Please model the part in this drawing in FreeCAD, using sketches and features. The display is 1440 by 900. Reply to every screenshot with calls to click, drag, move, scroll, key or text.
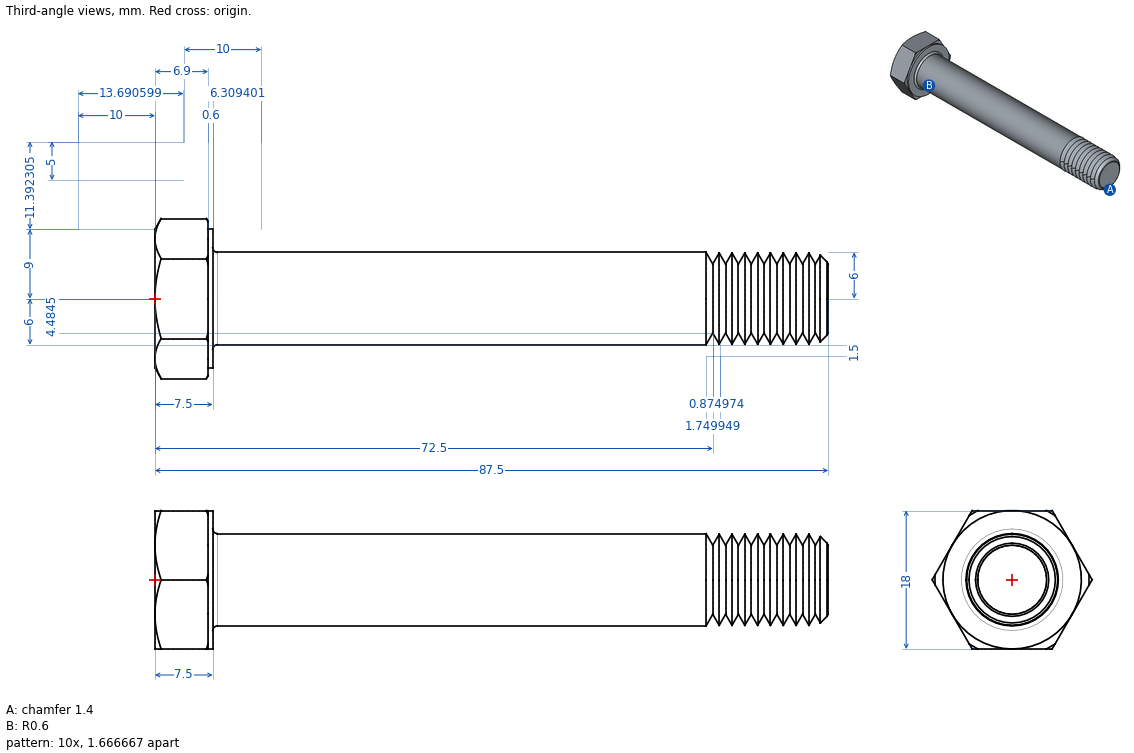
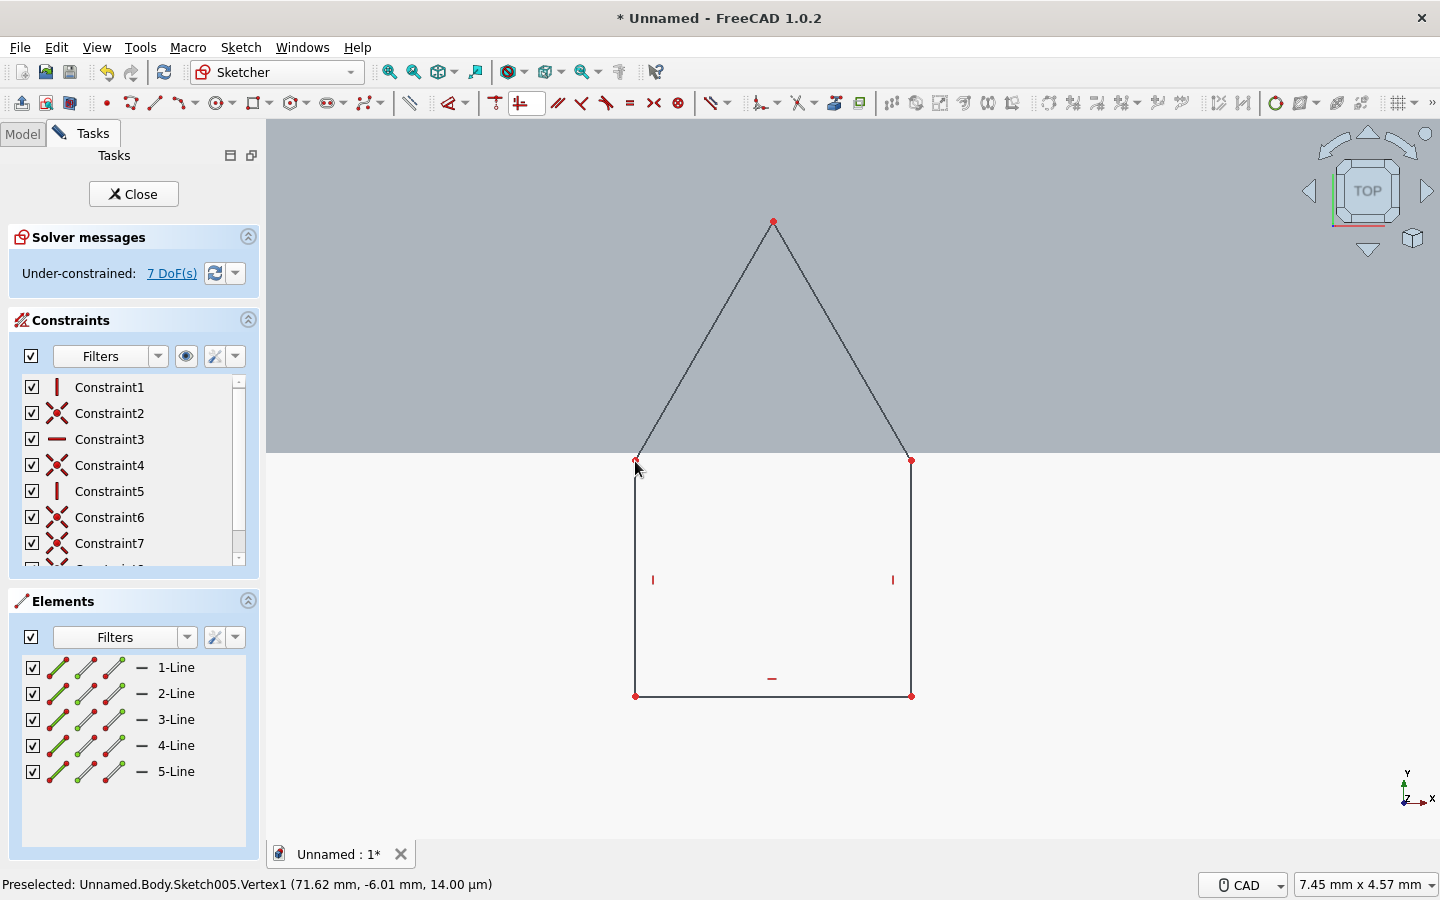
click(448, 104)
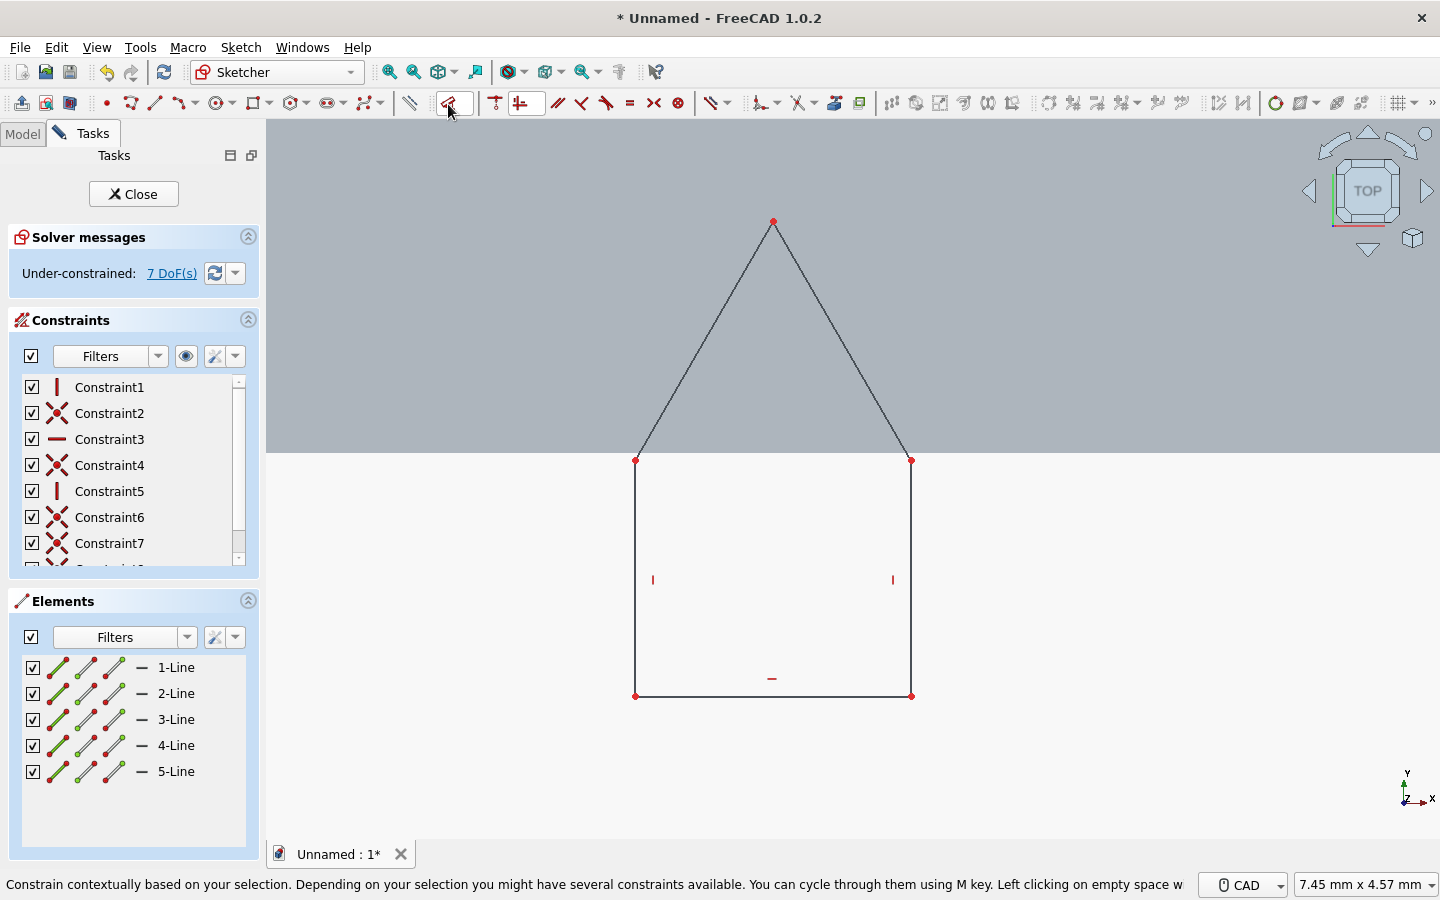
click(635, 461)
click(669, 304)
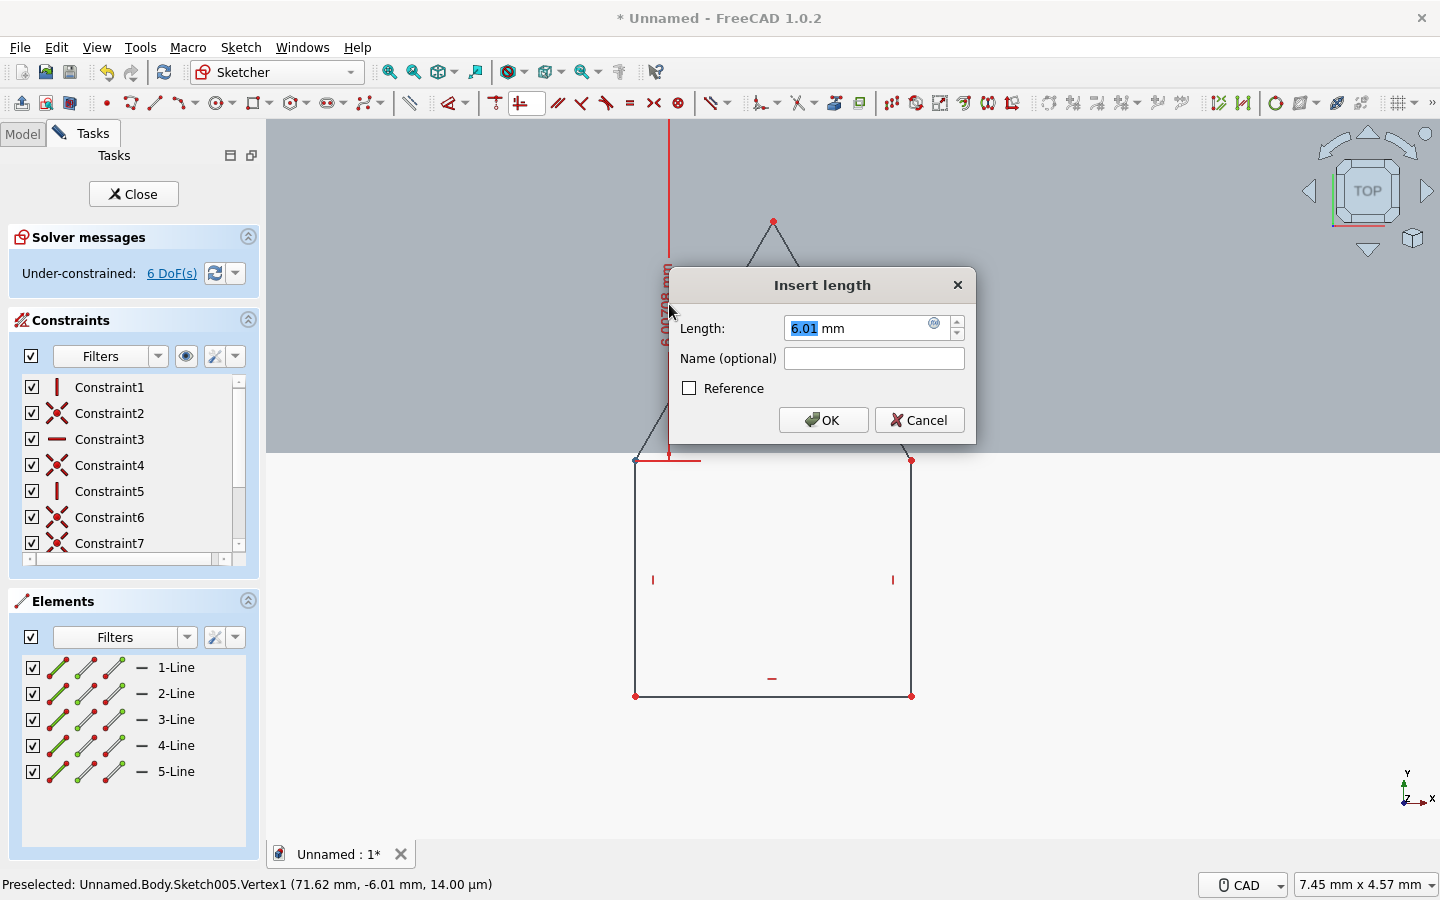
text(6)
key(Return)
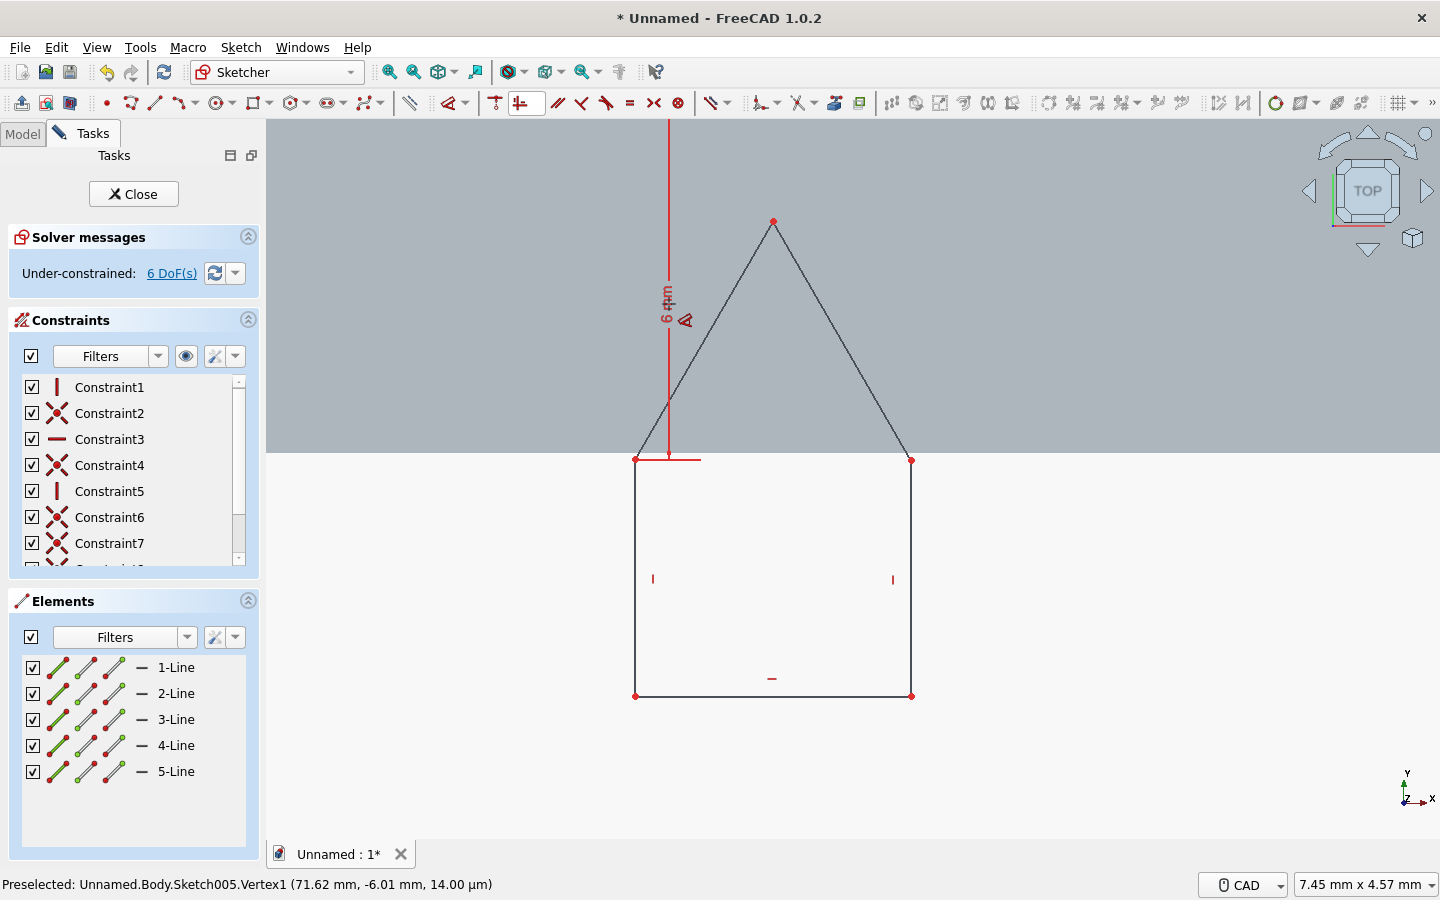
click(911, 461)
click(945, 304)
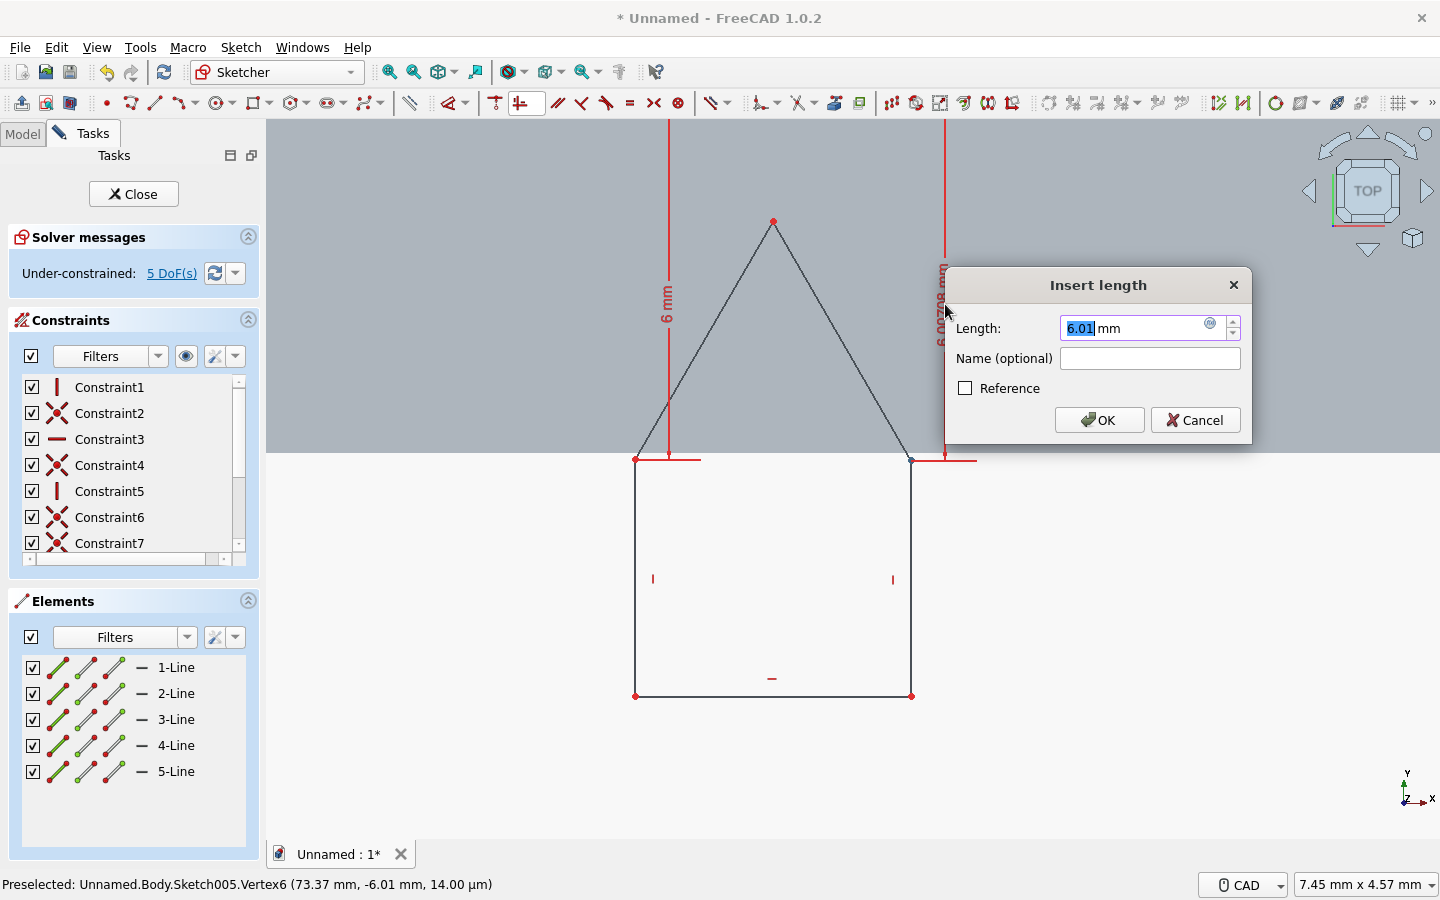
text(6)
key(Return)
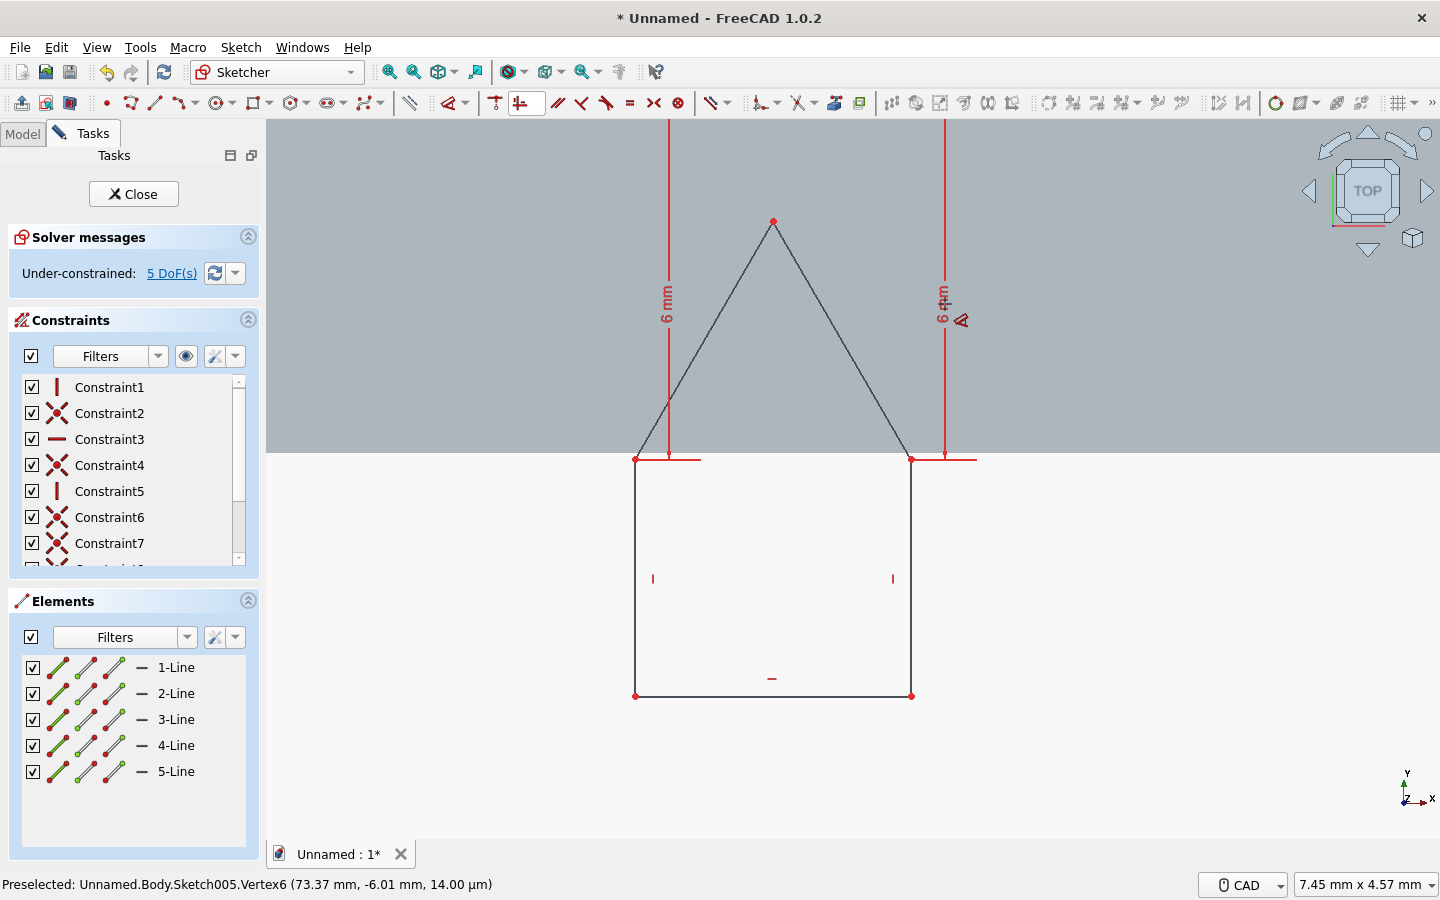
click(635, 531)
click(601, 578)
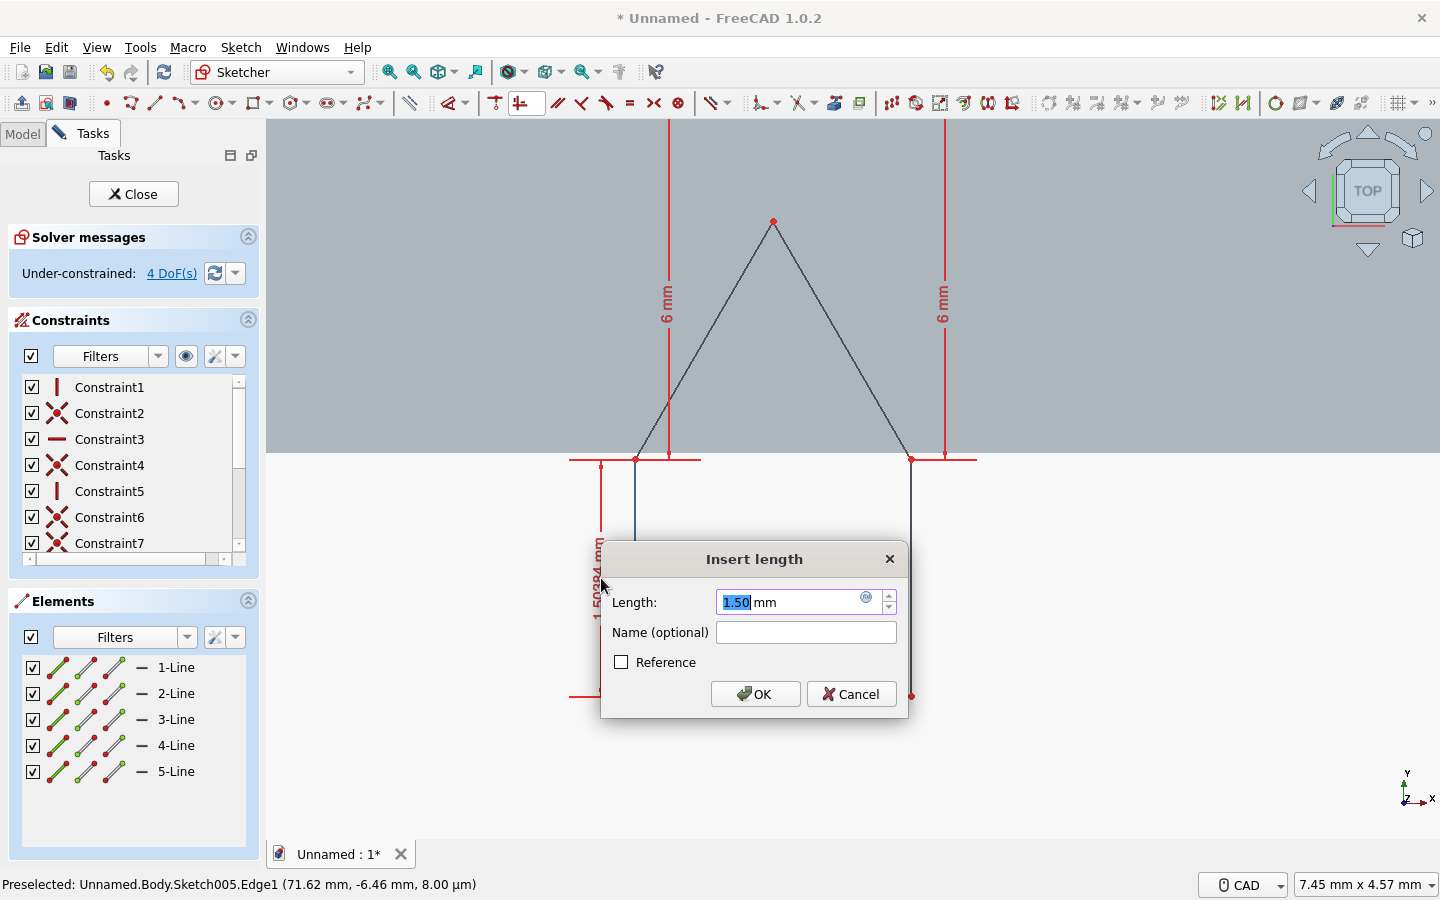
text(1.5)
key(Return)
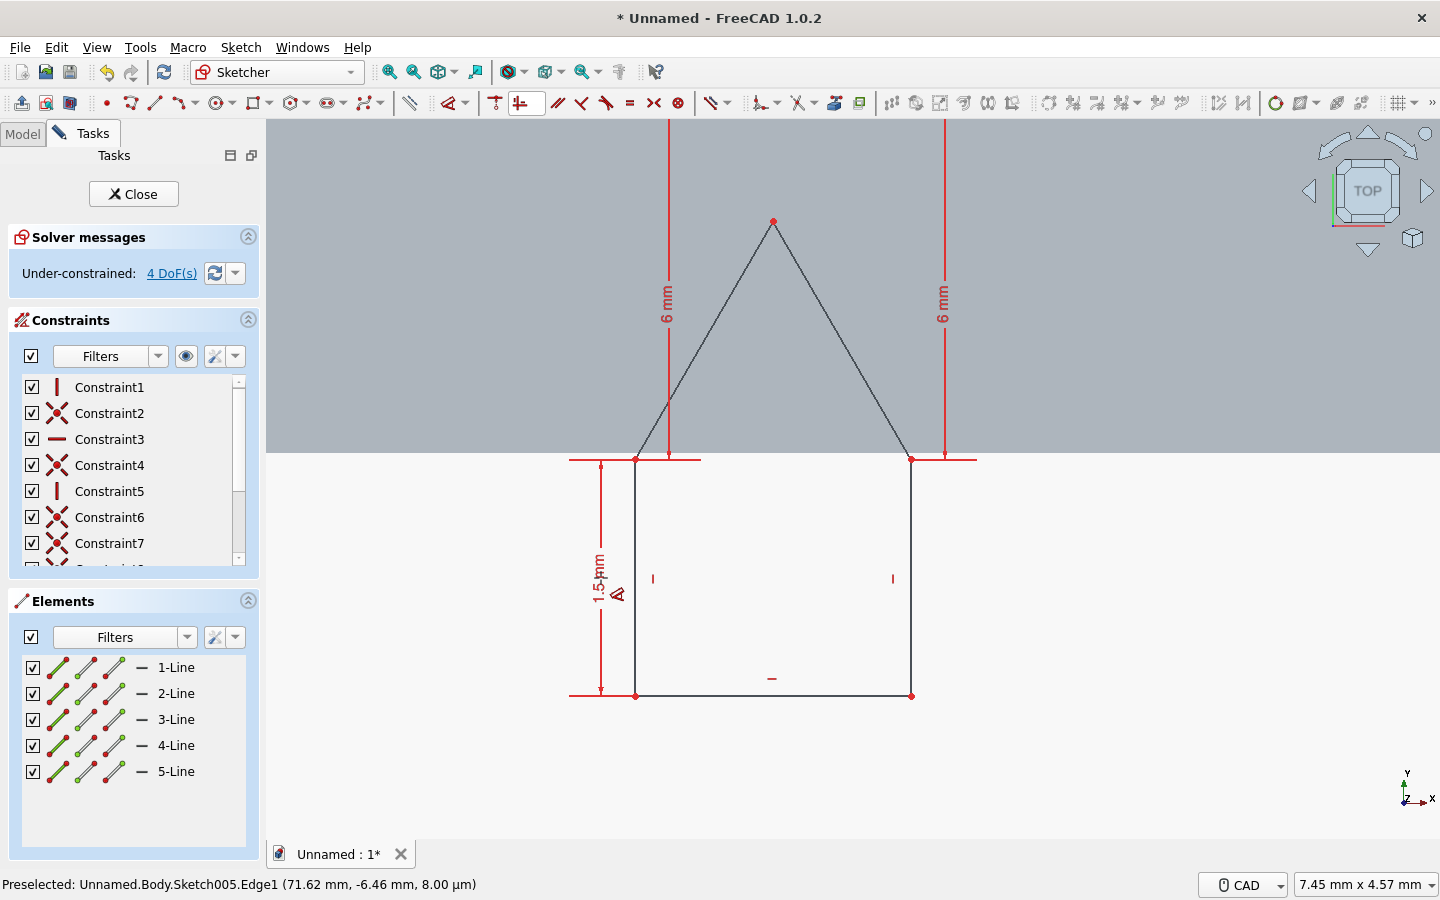
click(773, 222)
click(533, 256)